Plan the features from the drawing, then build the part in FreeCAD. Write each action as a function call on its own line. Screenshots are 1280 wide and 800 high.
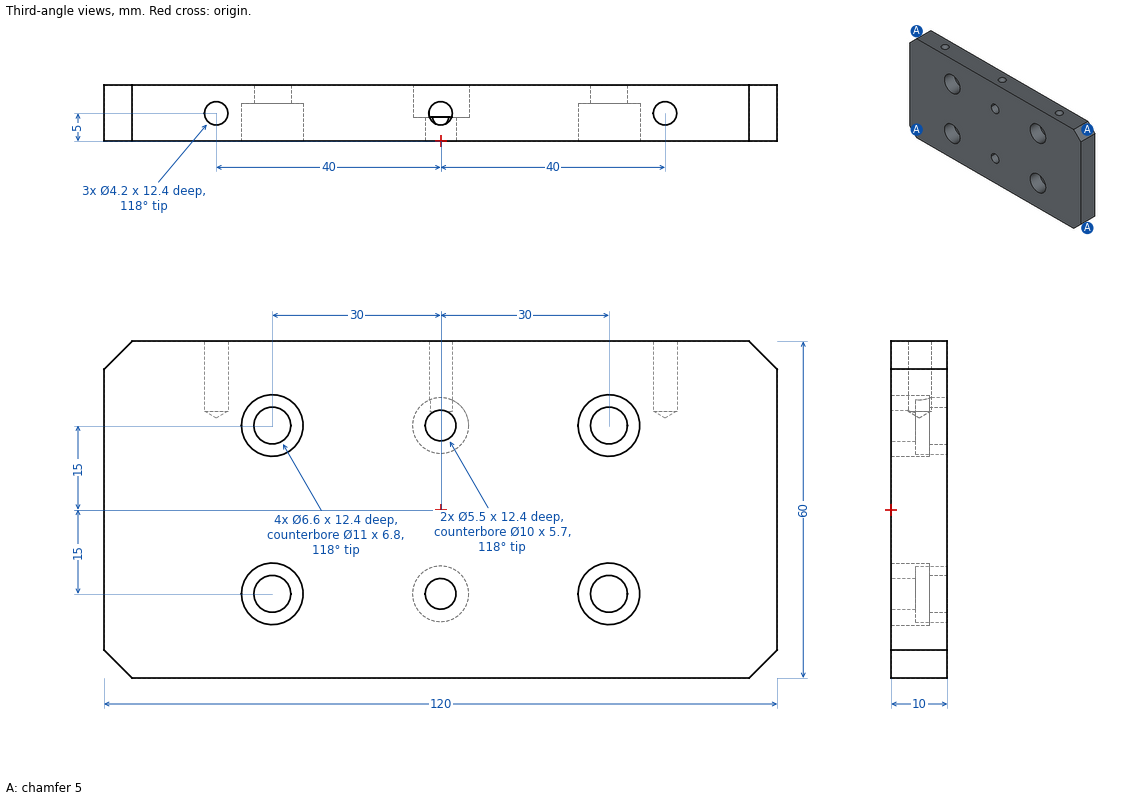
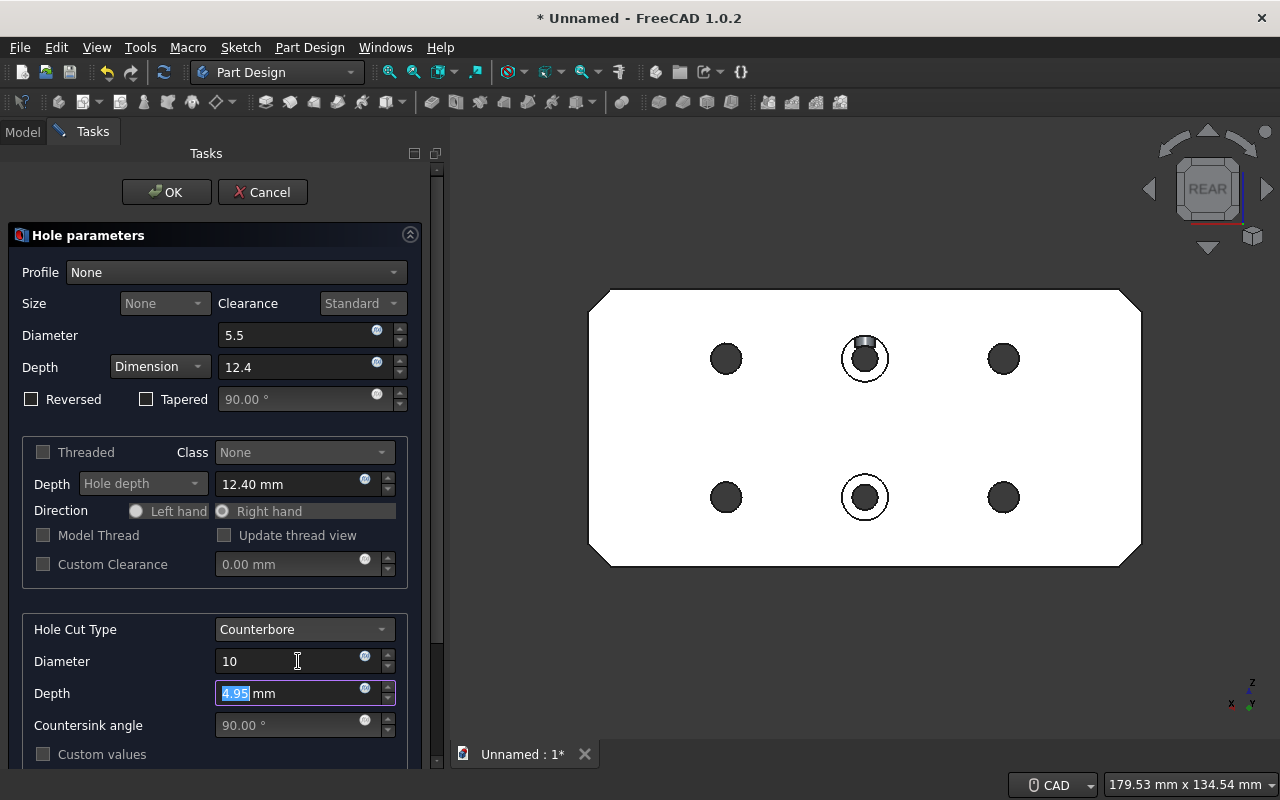
text(5.7)
key(Tab)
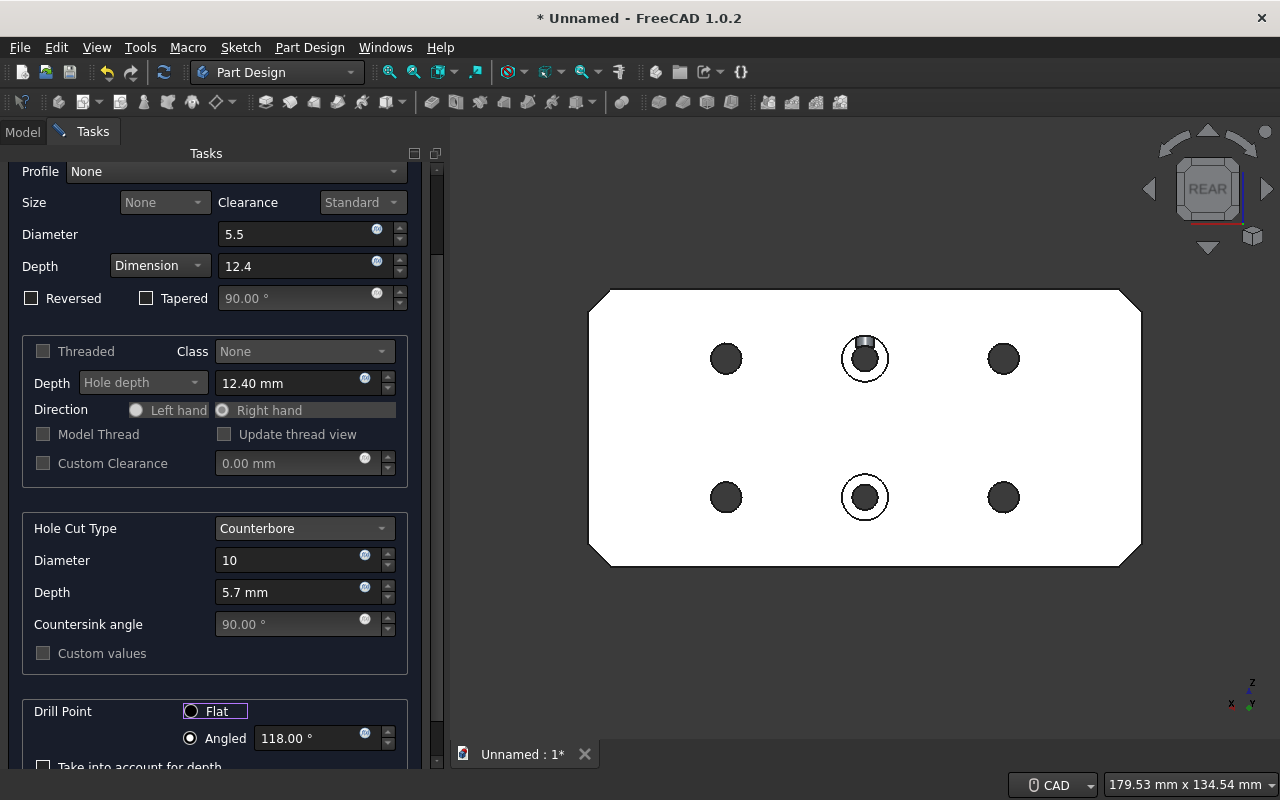
scroll(437, 466, up, 3)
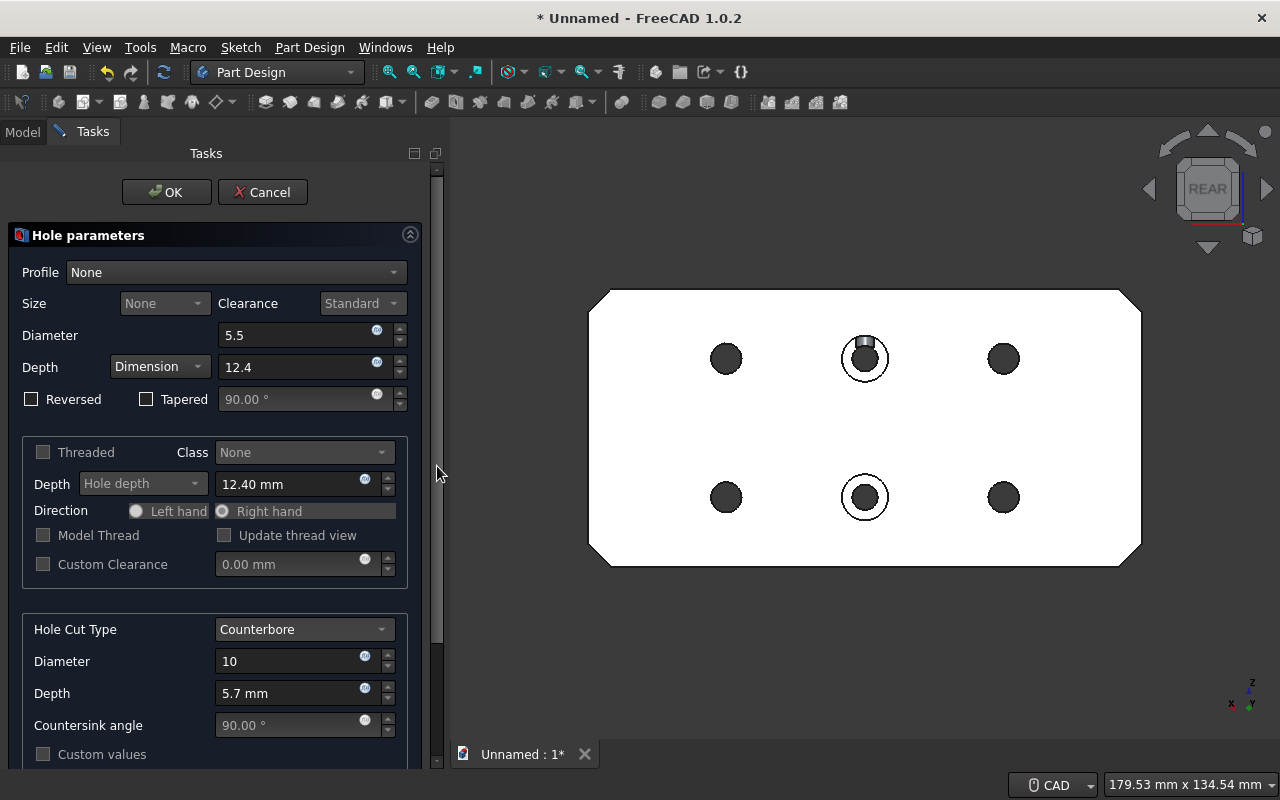
click(167, 192)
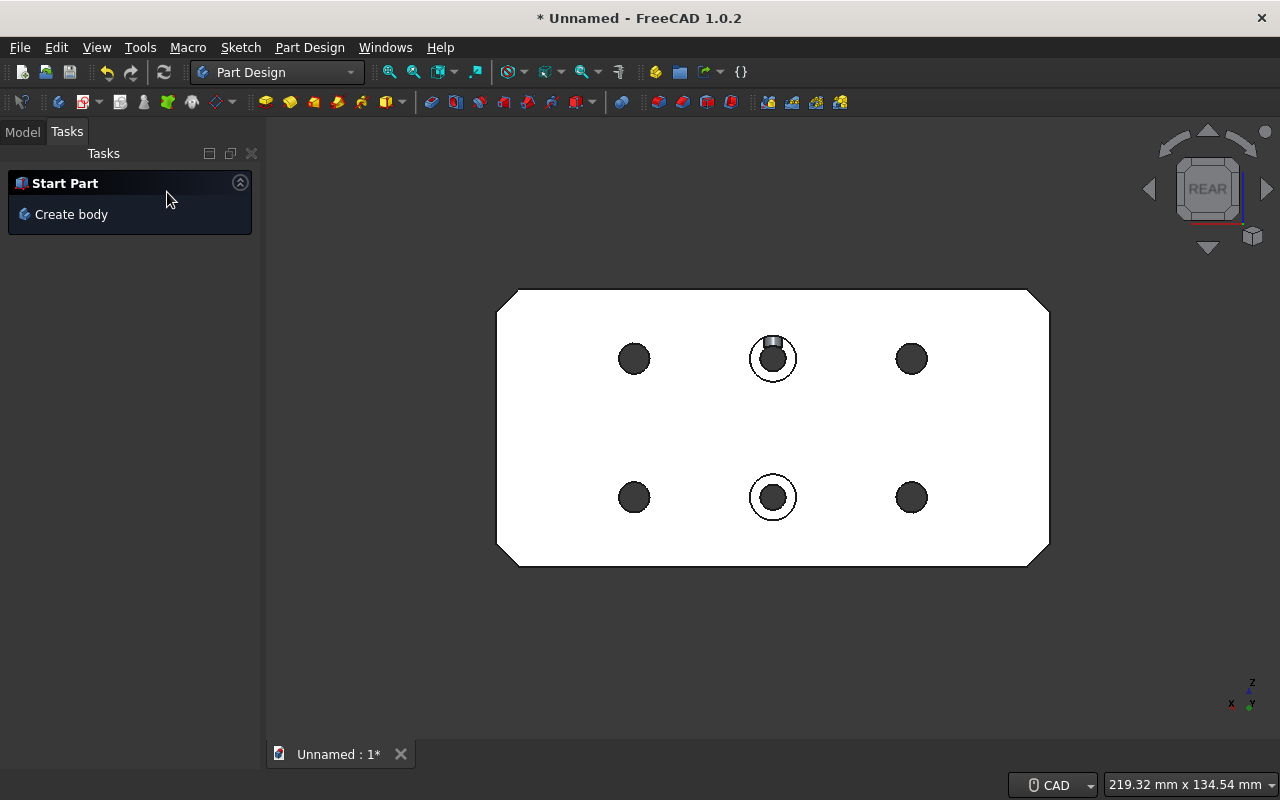
key(0)